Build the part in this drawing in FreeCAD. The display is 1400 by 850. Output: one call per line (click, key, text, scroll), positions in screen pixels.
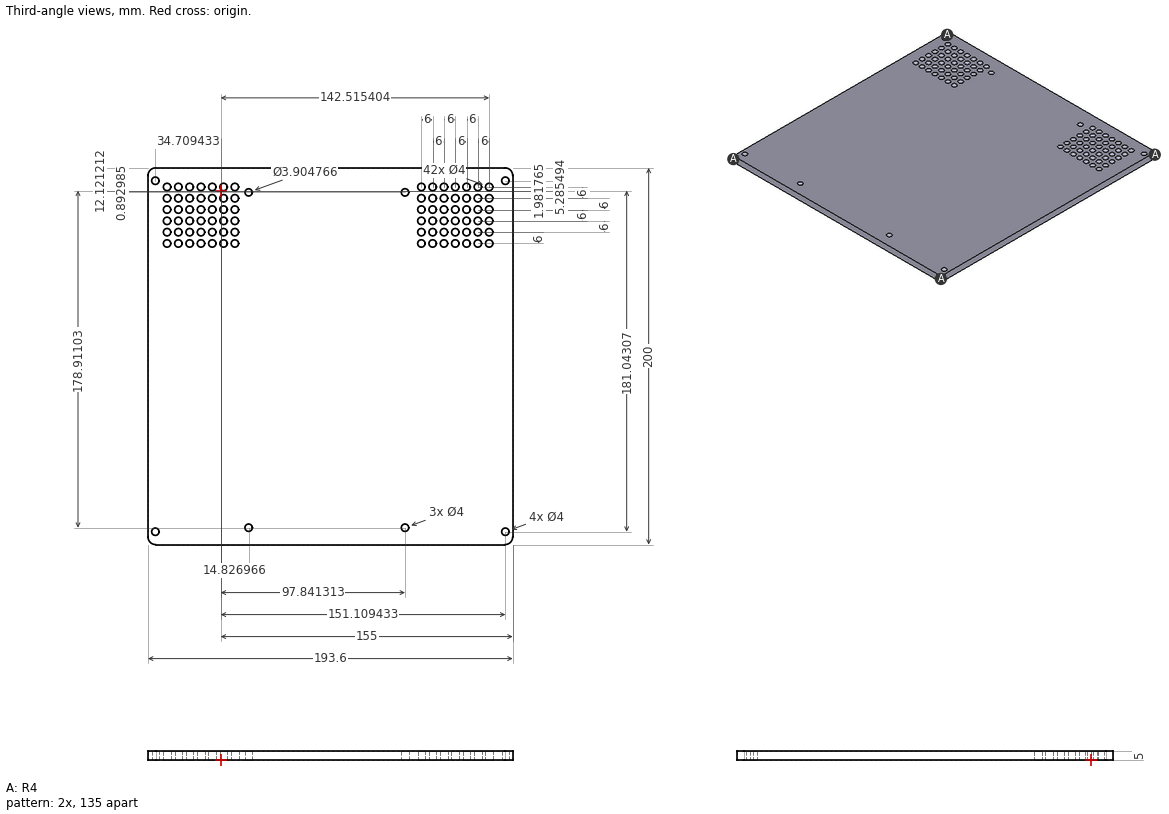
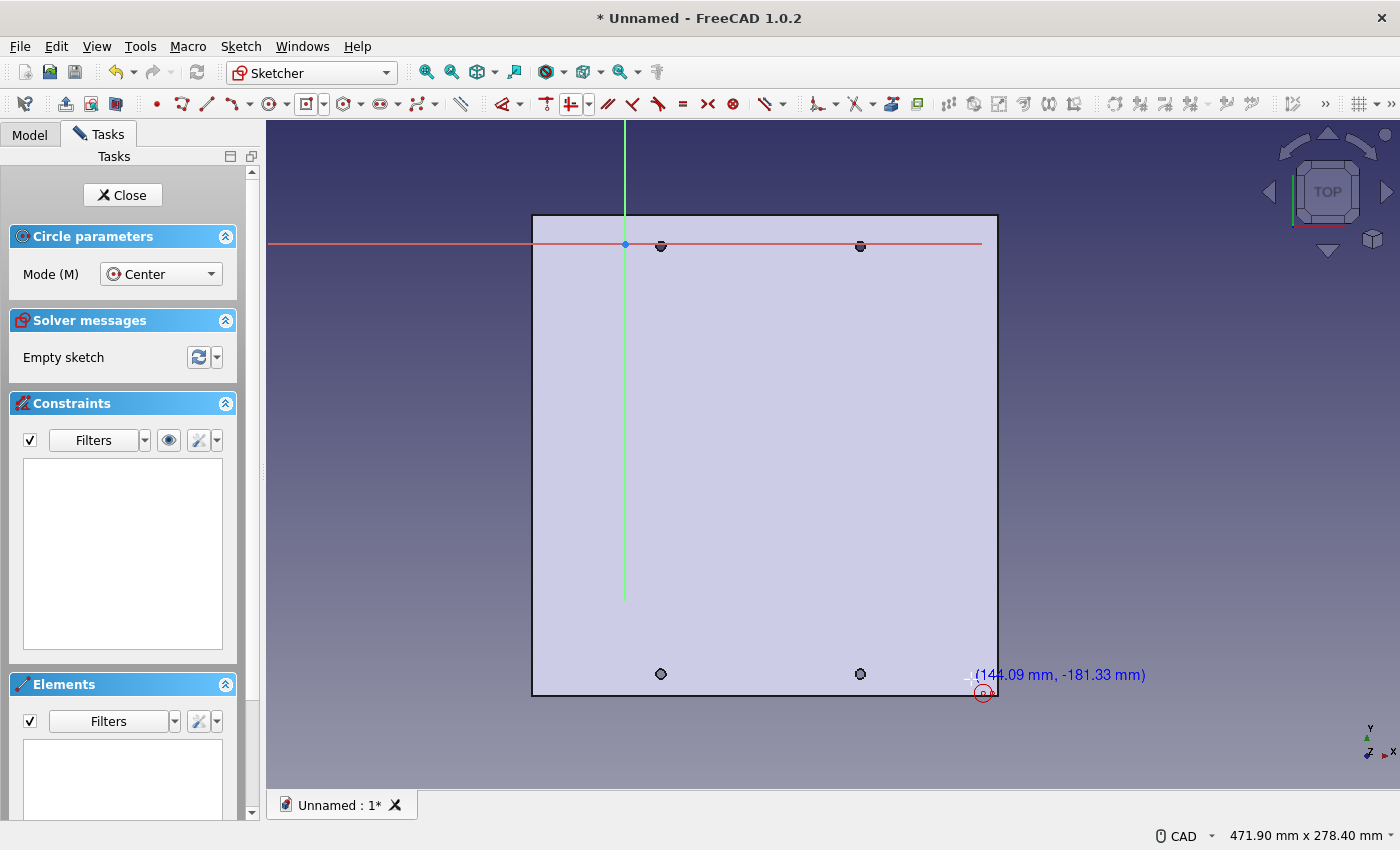
click(988, 679)
move(992, 676)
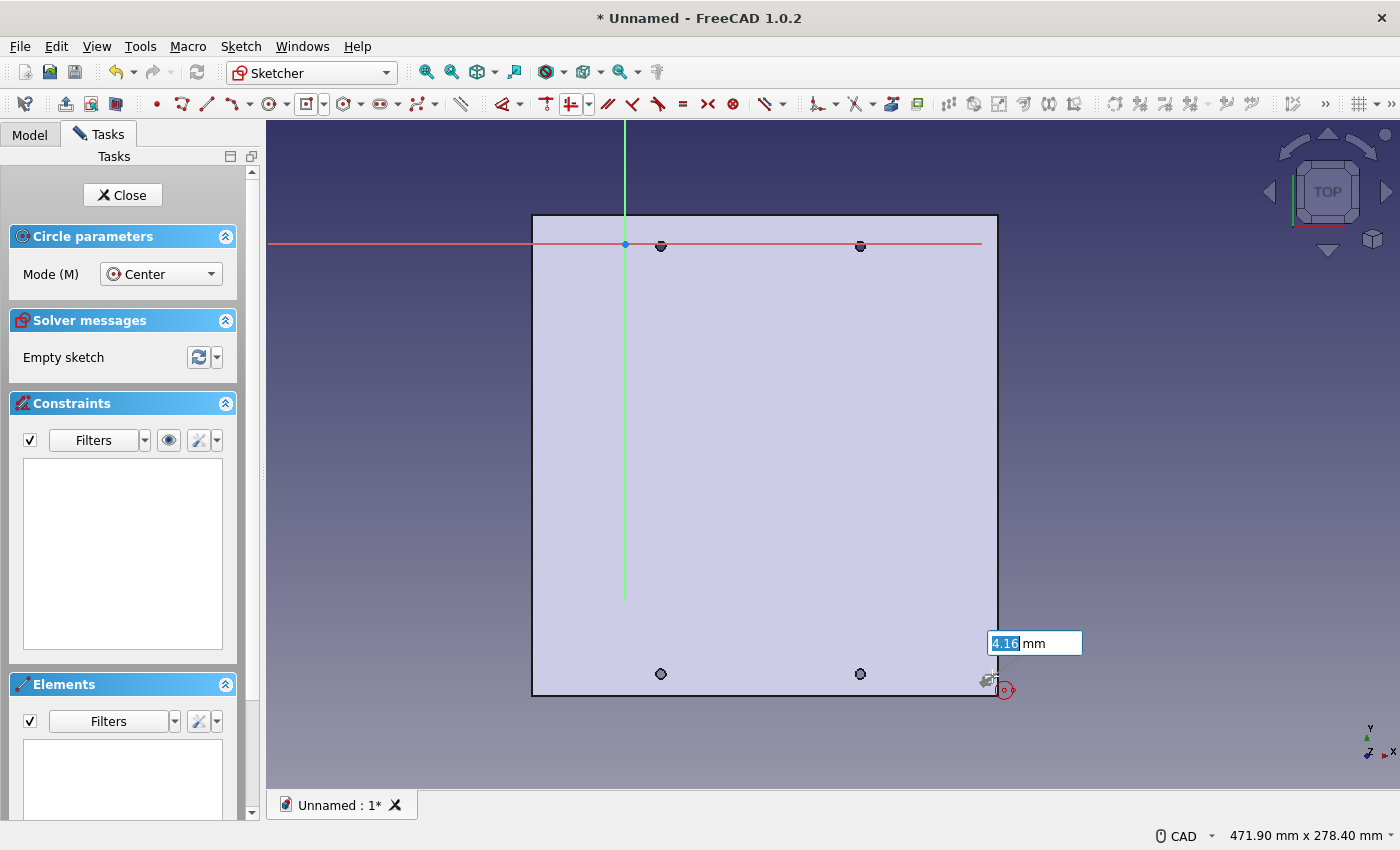
text(4)
key(Return)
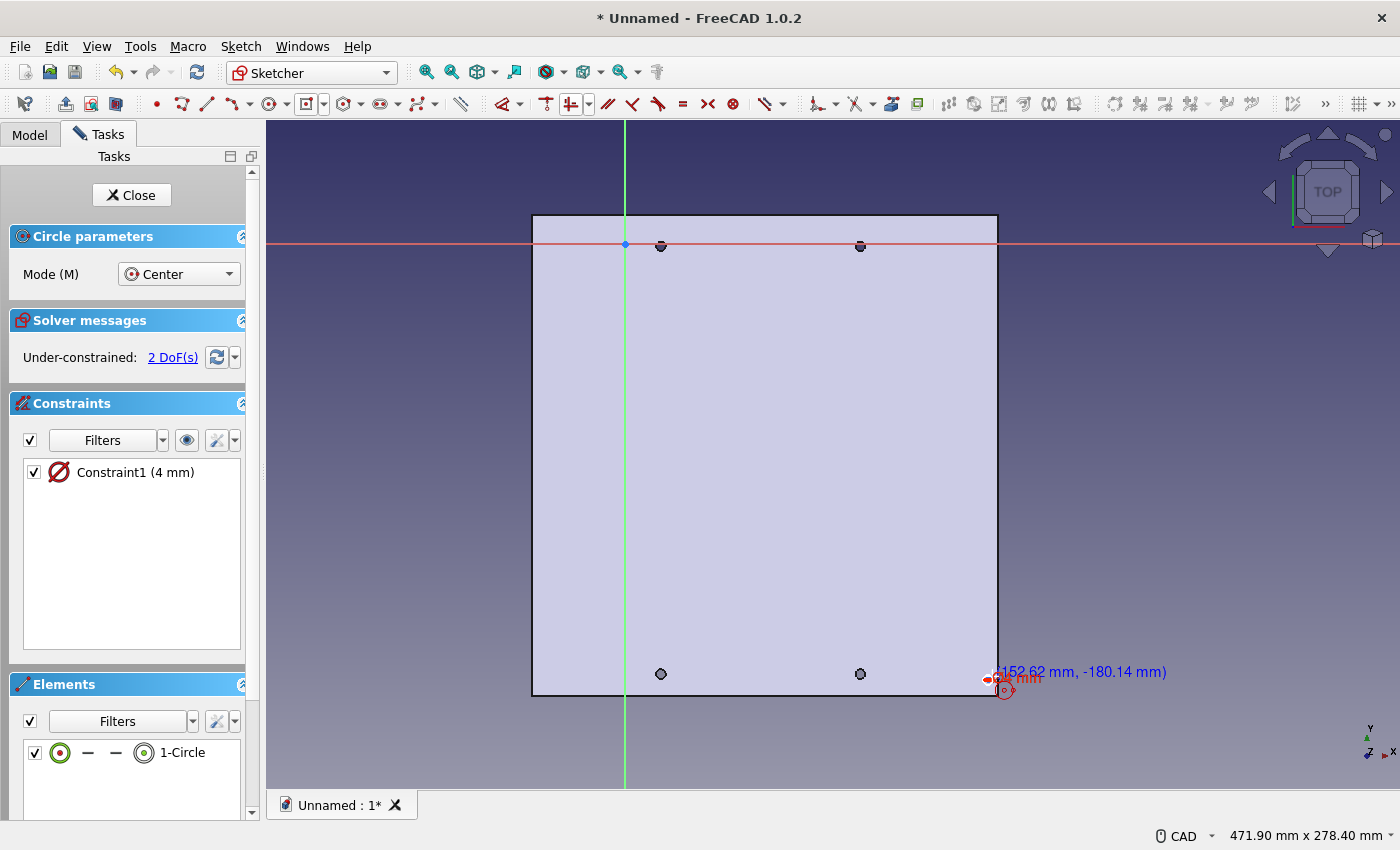
scroll(988, 231, up, 8)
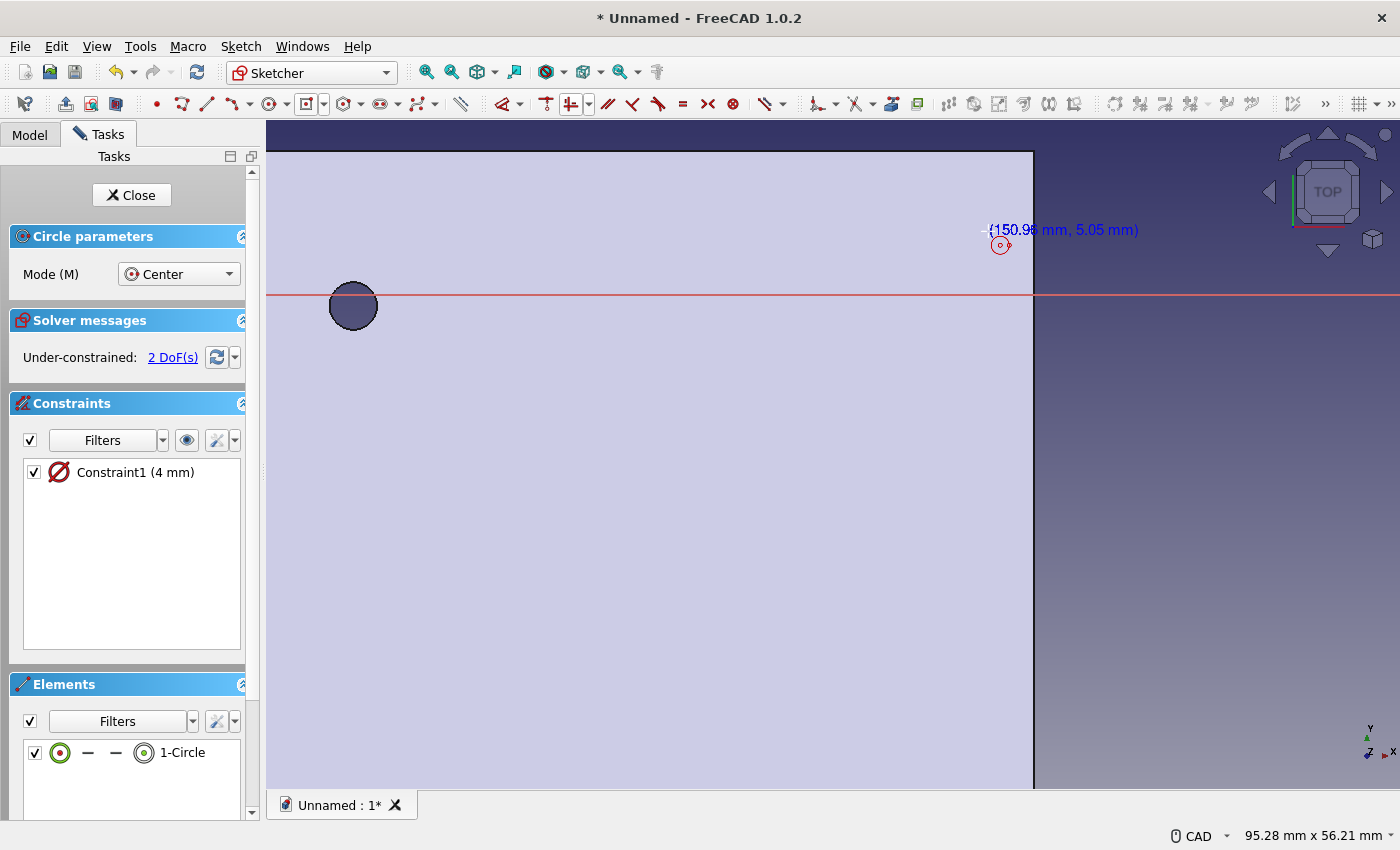
scroll(988, 230, down, 8)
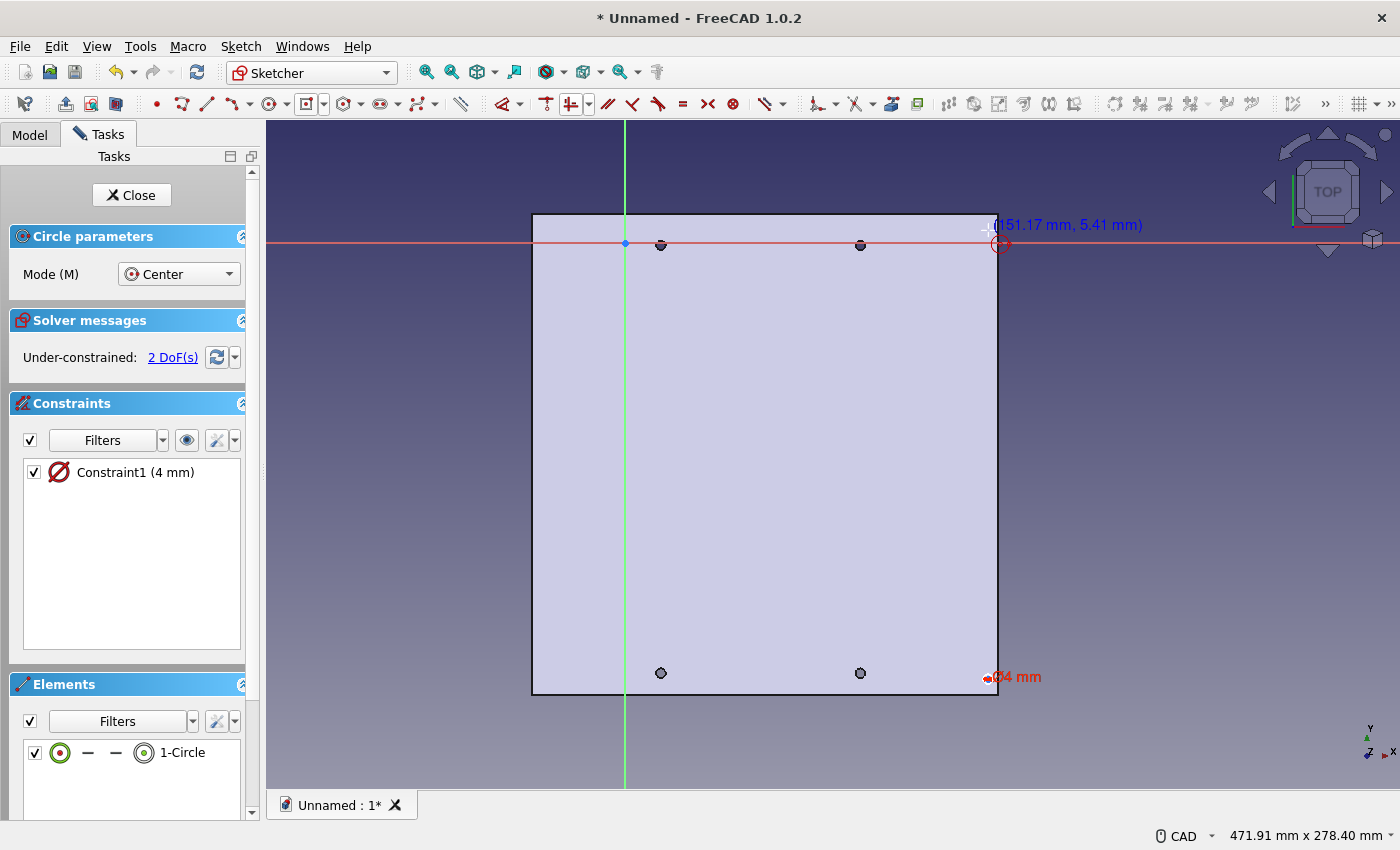
scroll(988, 231, up, 2)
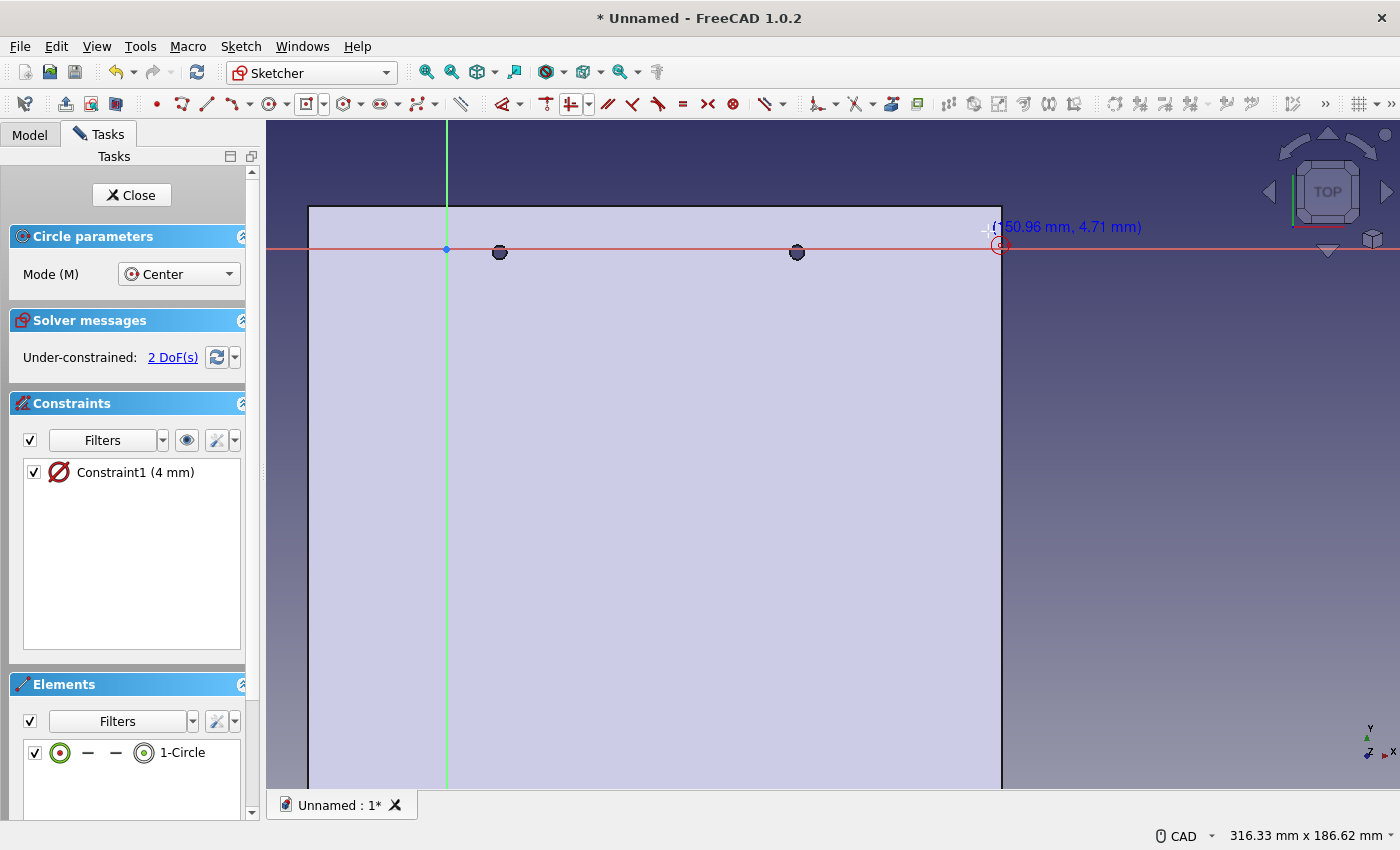
click(988, 230)
move(993, 225)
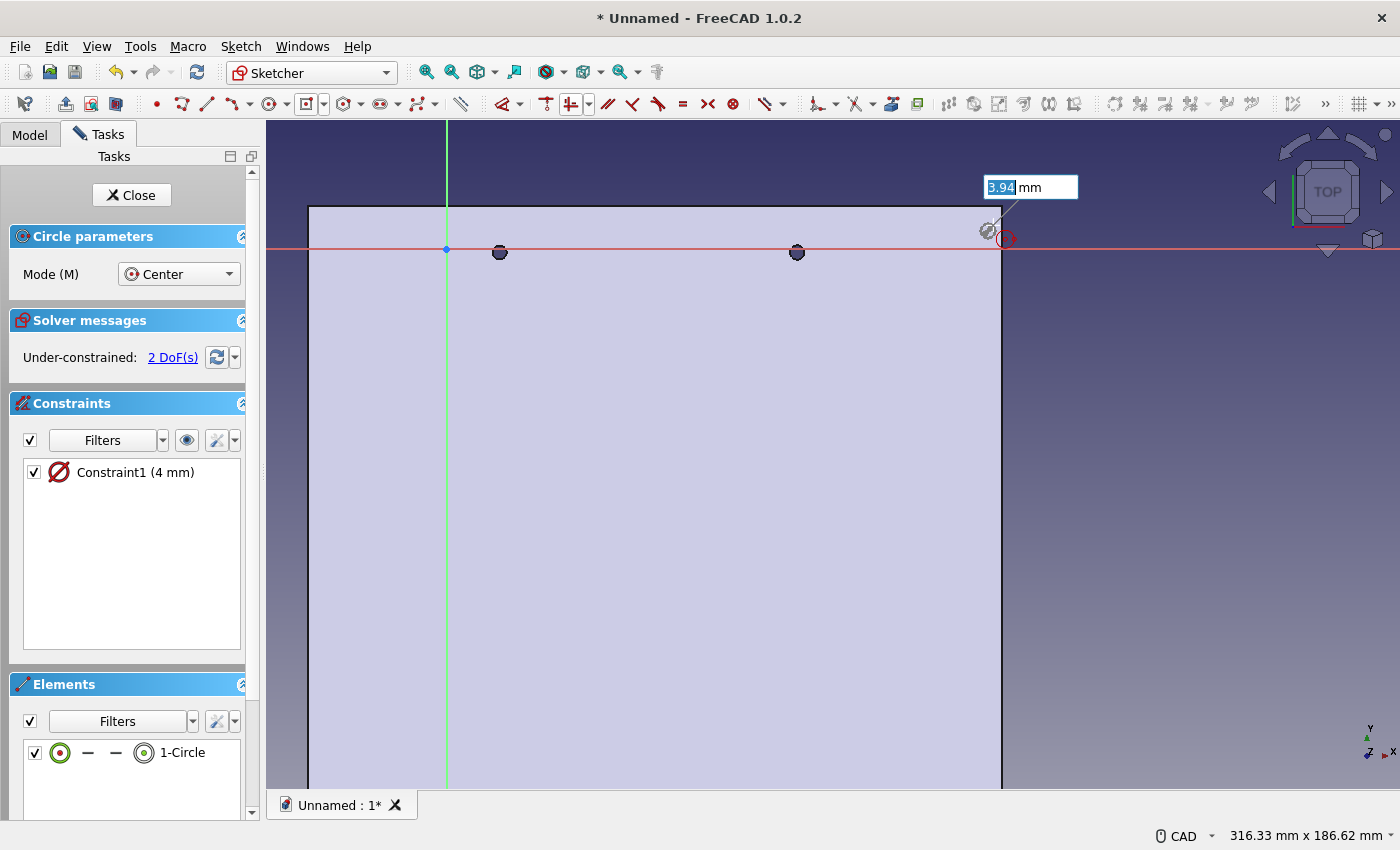
text(4)
key(Return)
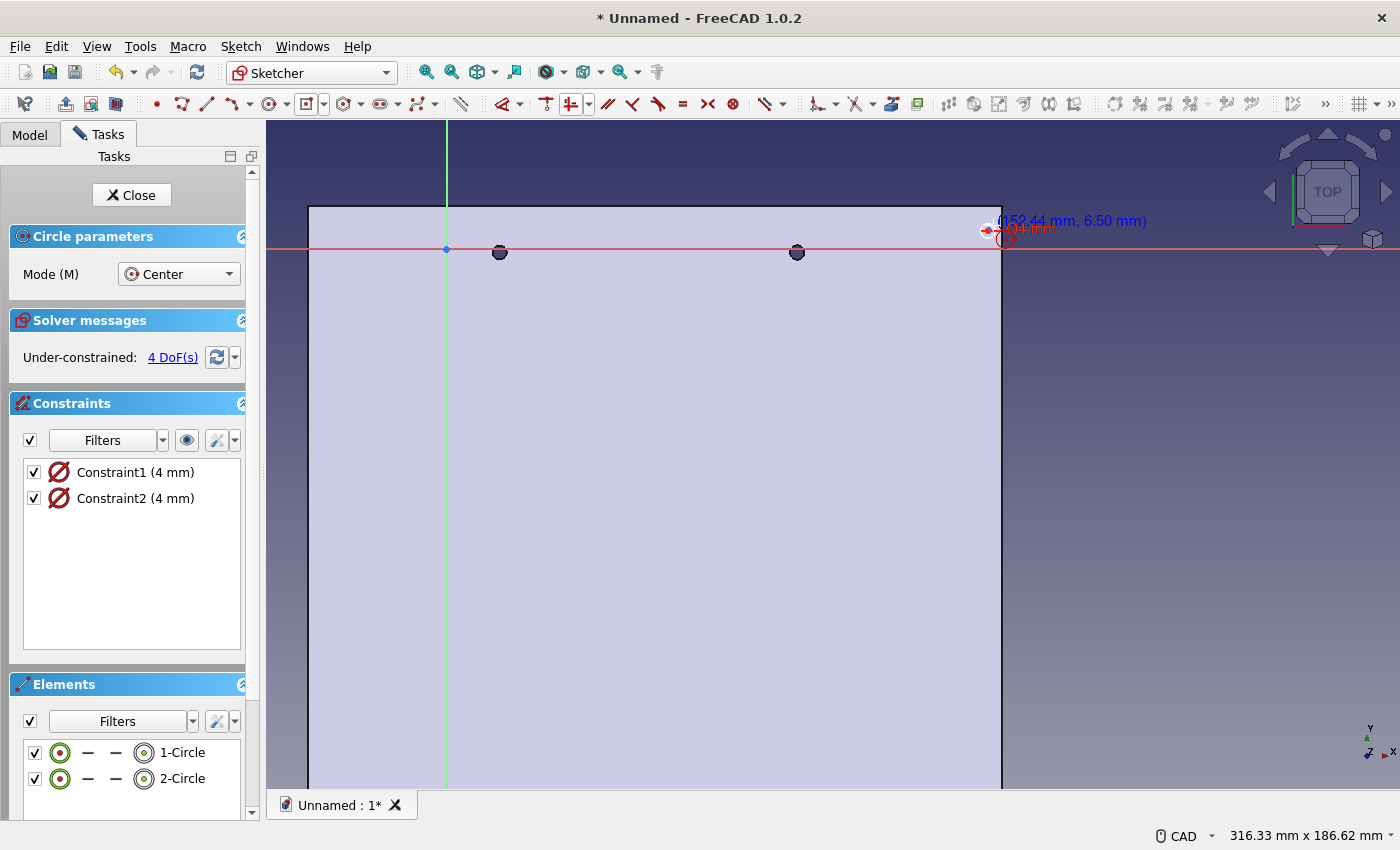
scroll(322, 230, up, 6)